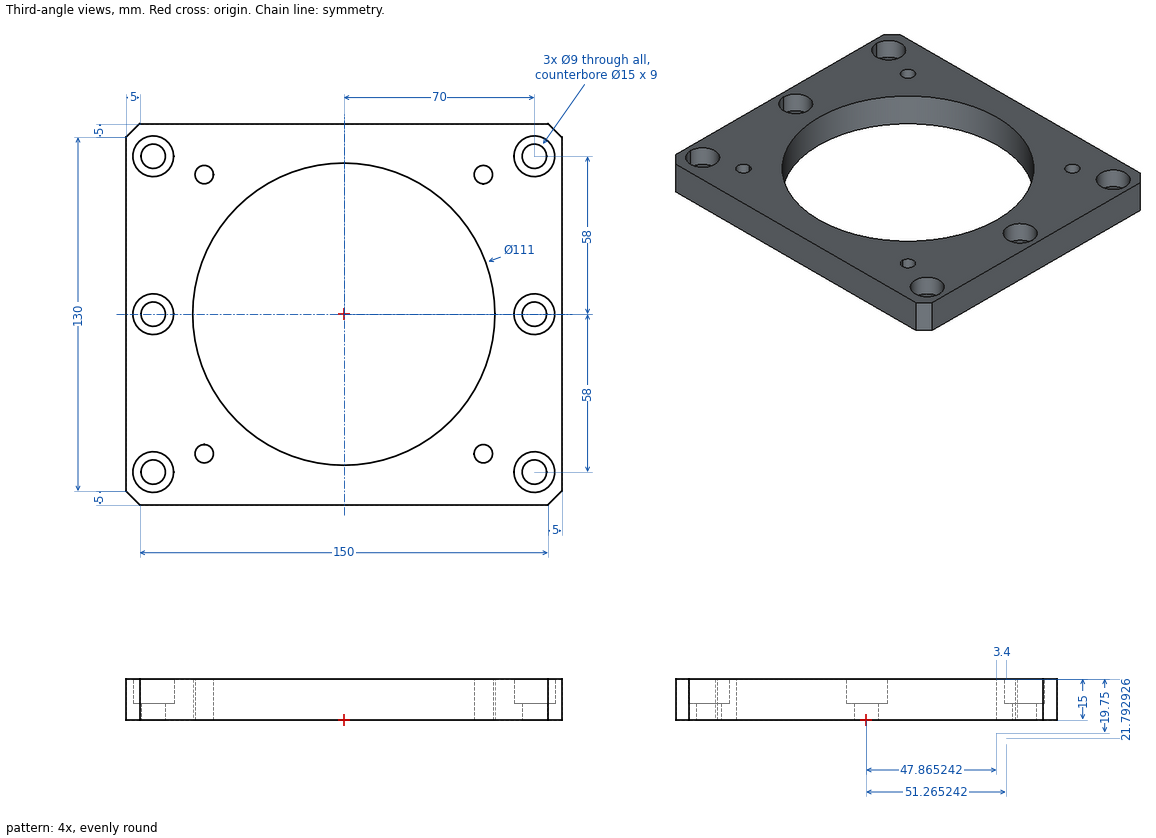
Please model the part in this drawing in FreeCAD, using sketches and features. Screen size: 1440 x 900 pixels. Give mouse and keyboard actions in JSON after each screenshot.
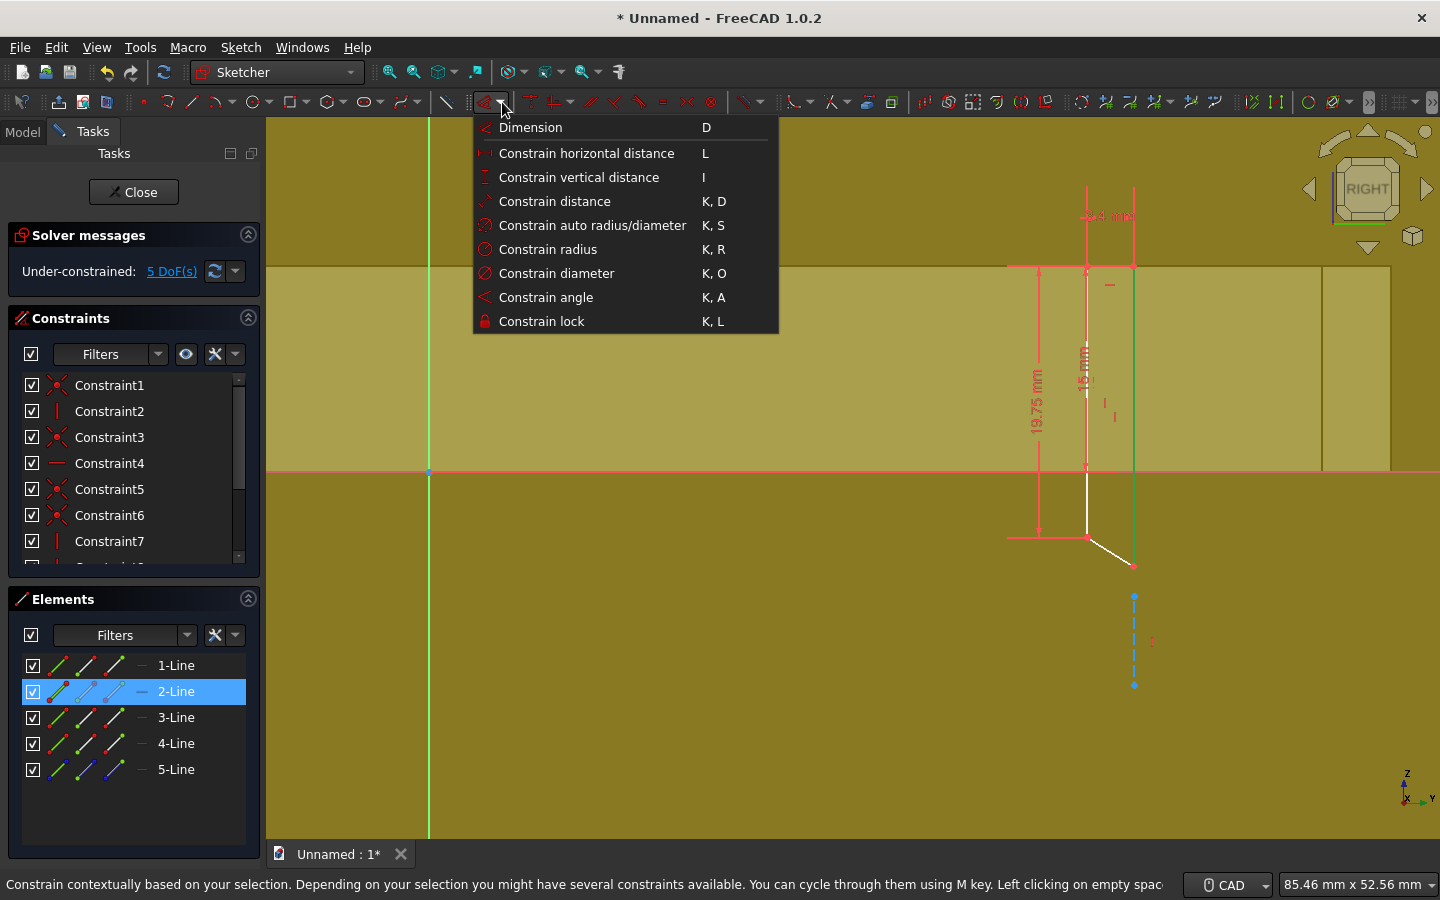
{"action": "left_click", "coordinate": [626, 177]}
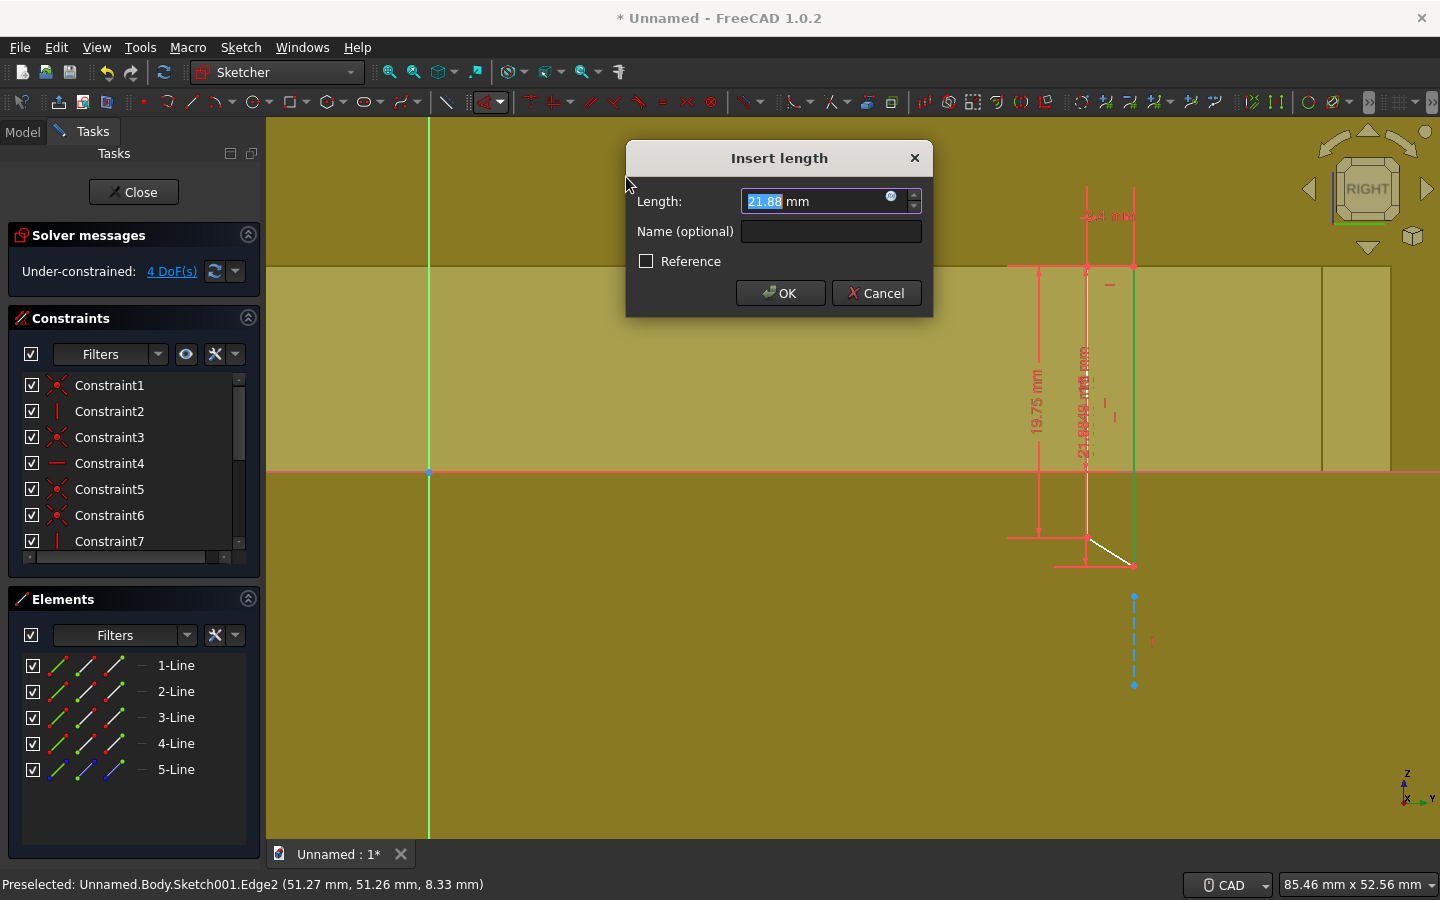
{"action": "type", "text": "21.792926"}
{"action": "key", "text": "Return"}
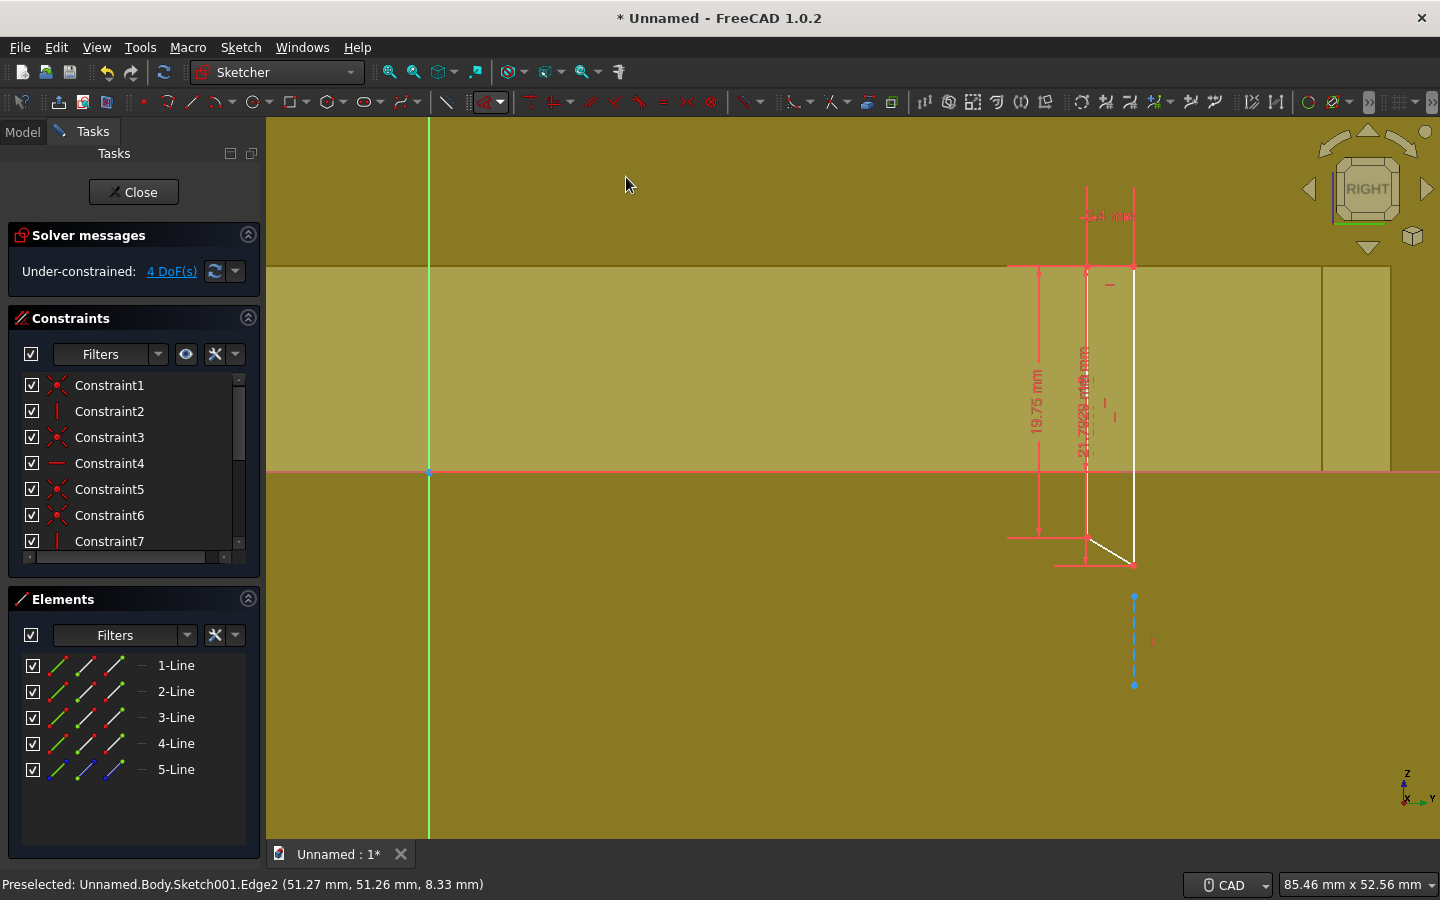
{"action": "left_click", "coordinate": [1087, 538]}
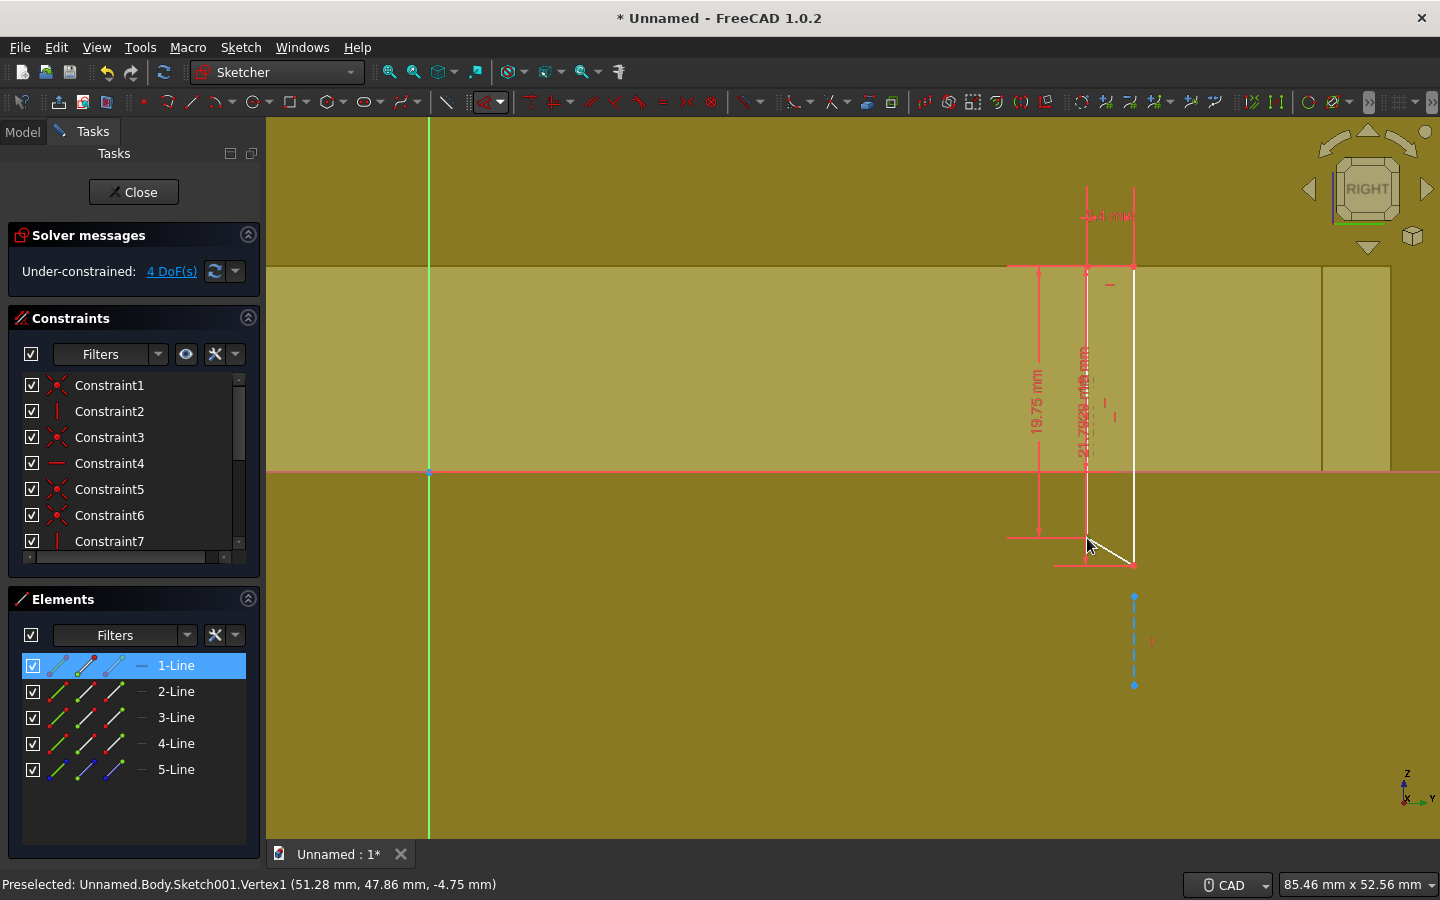
{"action": "key", "text": "l"}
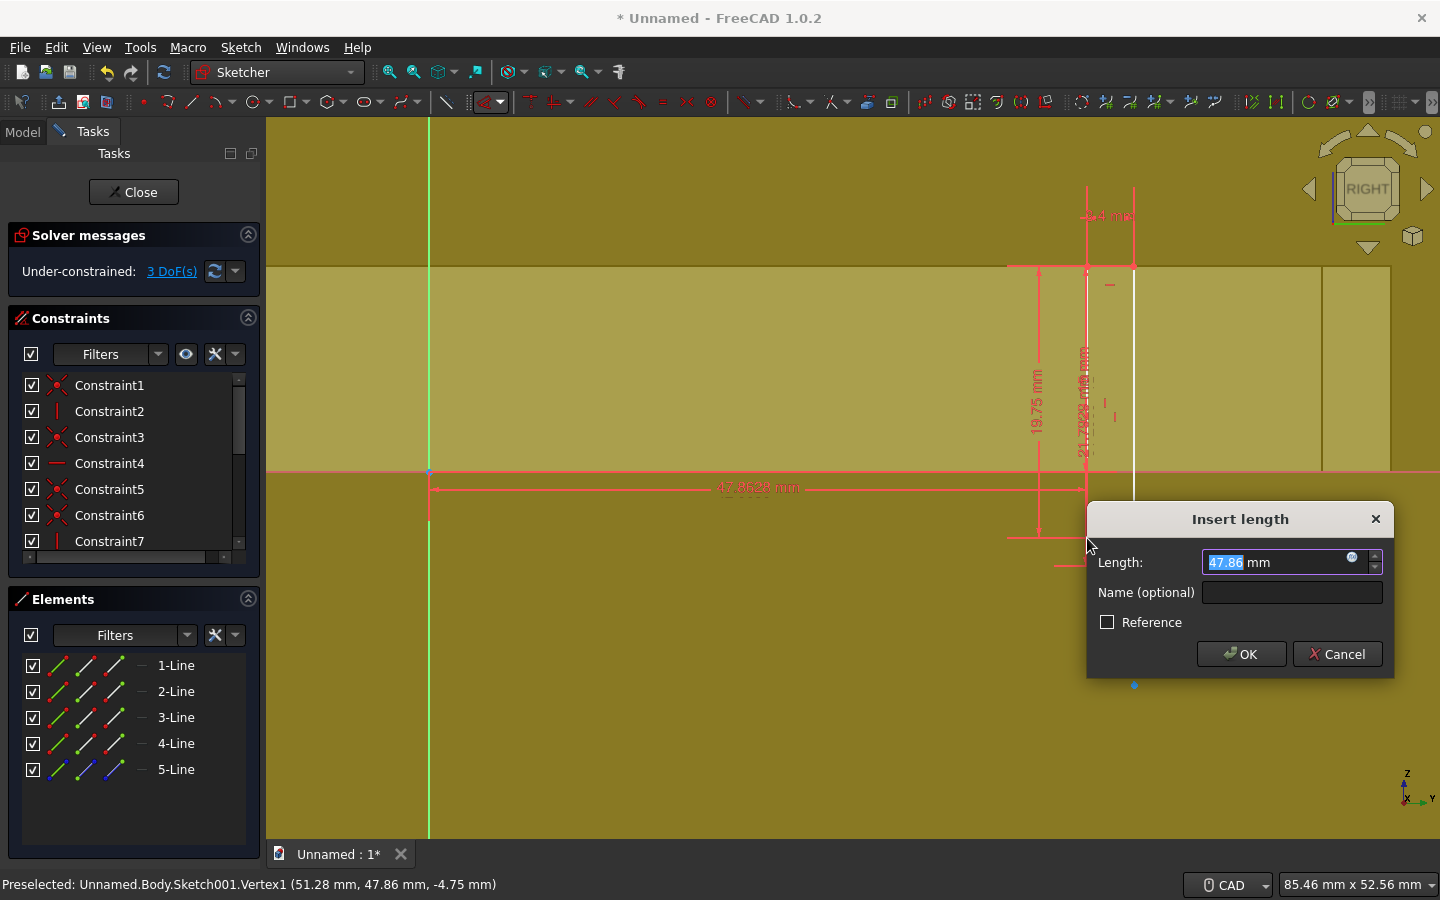
{"action": "type", "text": "47.865242"}
{"action": "key", "text": "Return"}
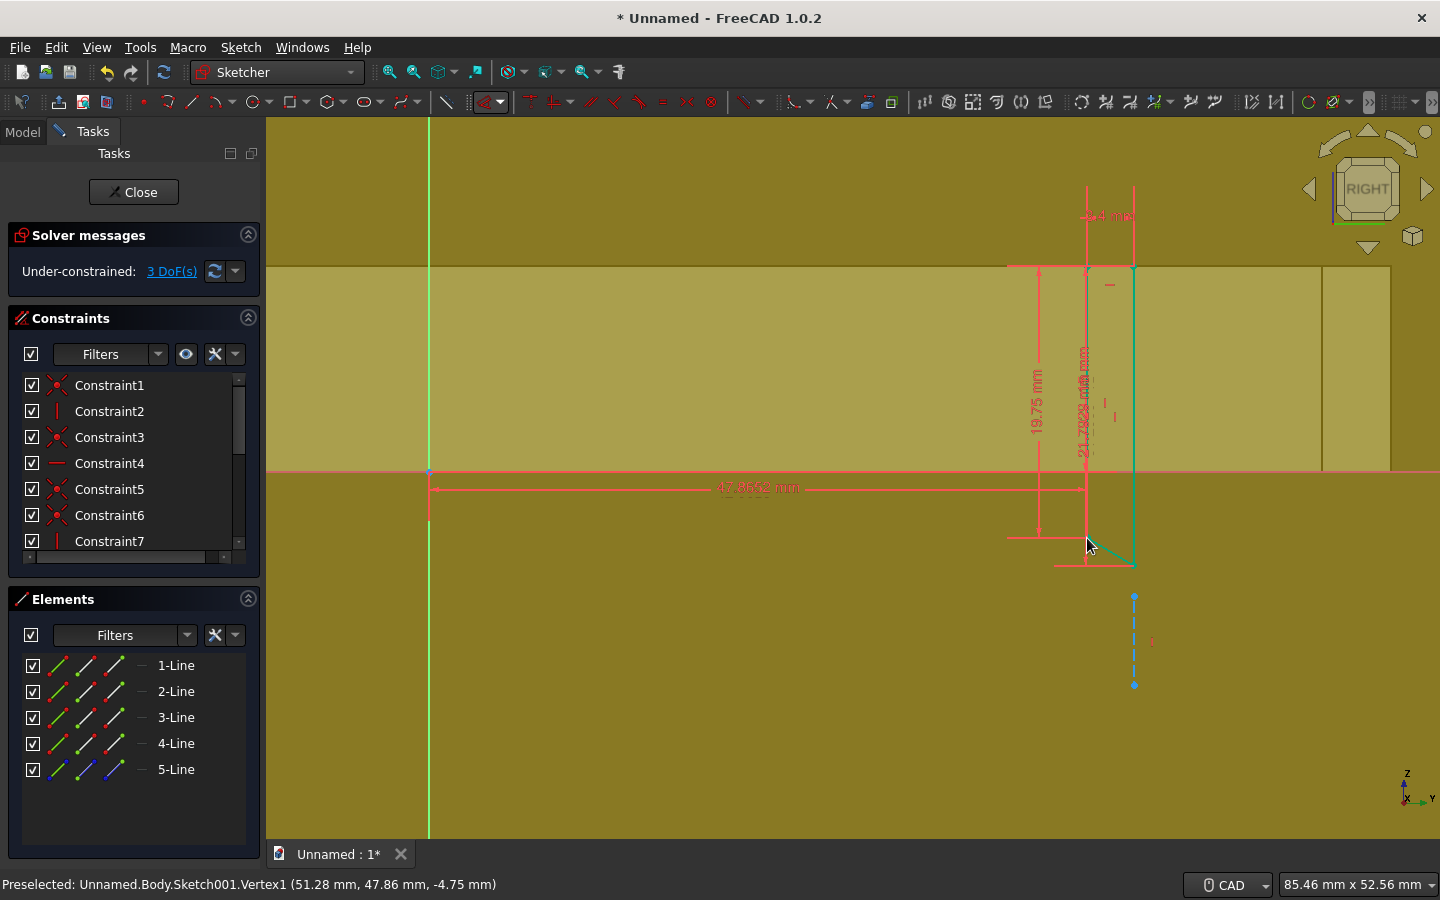
{"action": "left_click", "coordinate": [1134, 597]}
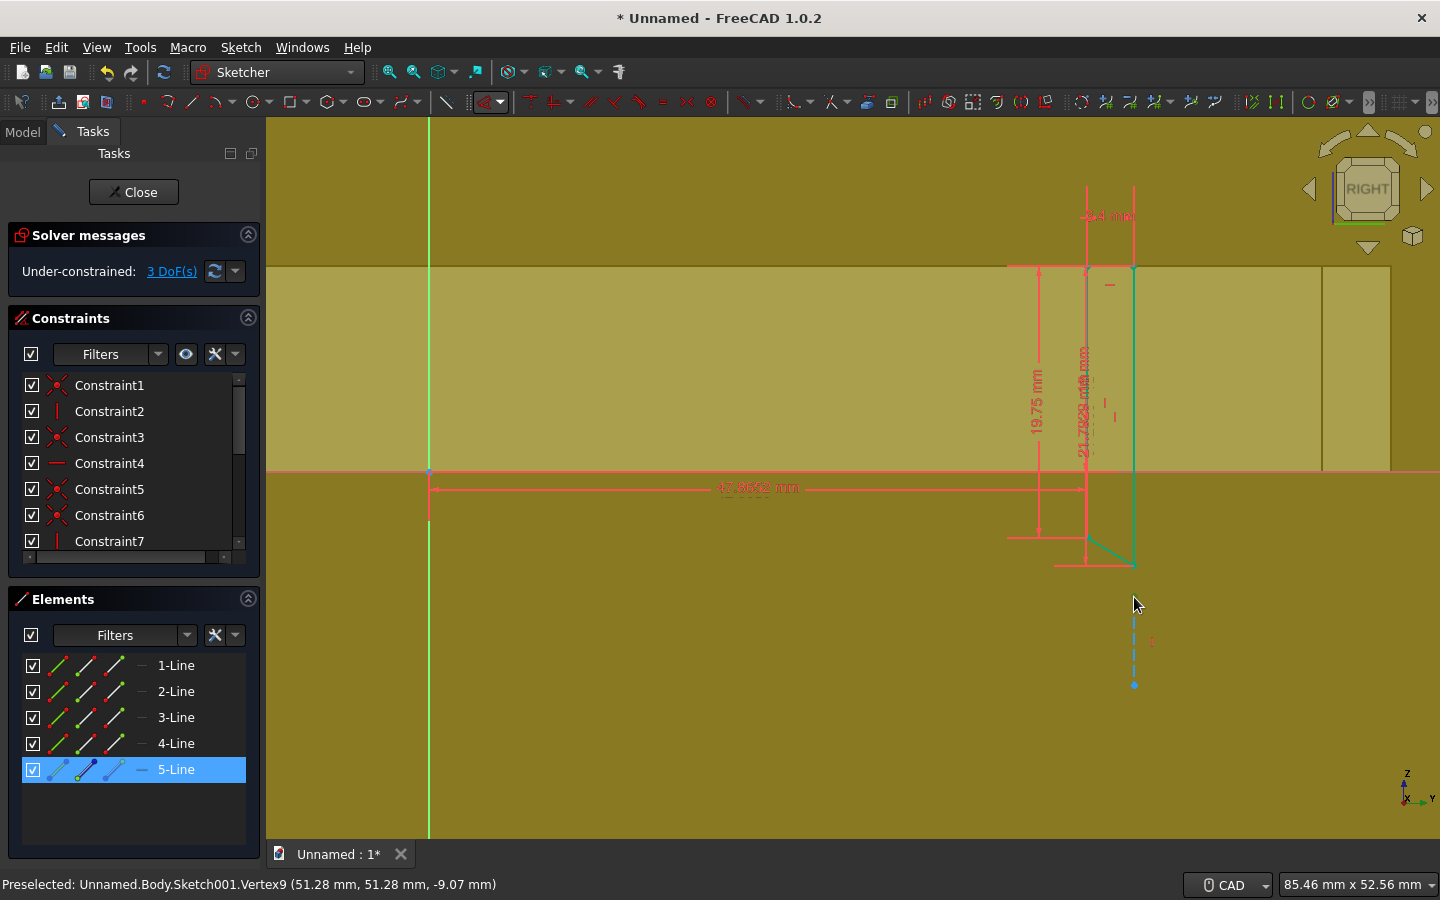
{"action": "key", "text": "l"}